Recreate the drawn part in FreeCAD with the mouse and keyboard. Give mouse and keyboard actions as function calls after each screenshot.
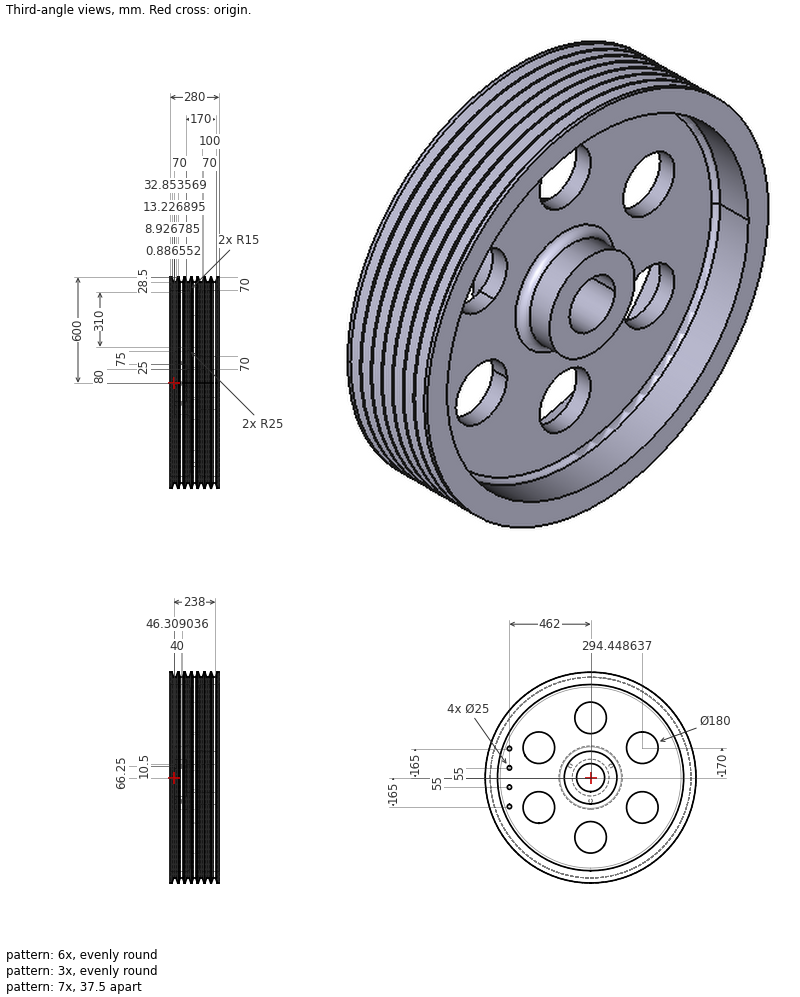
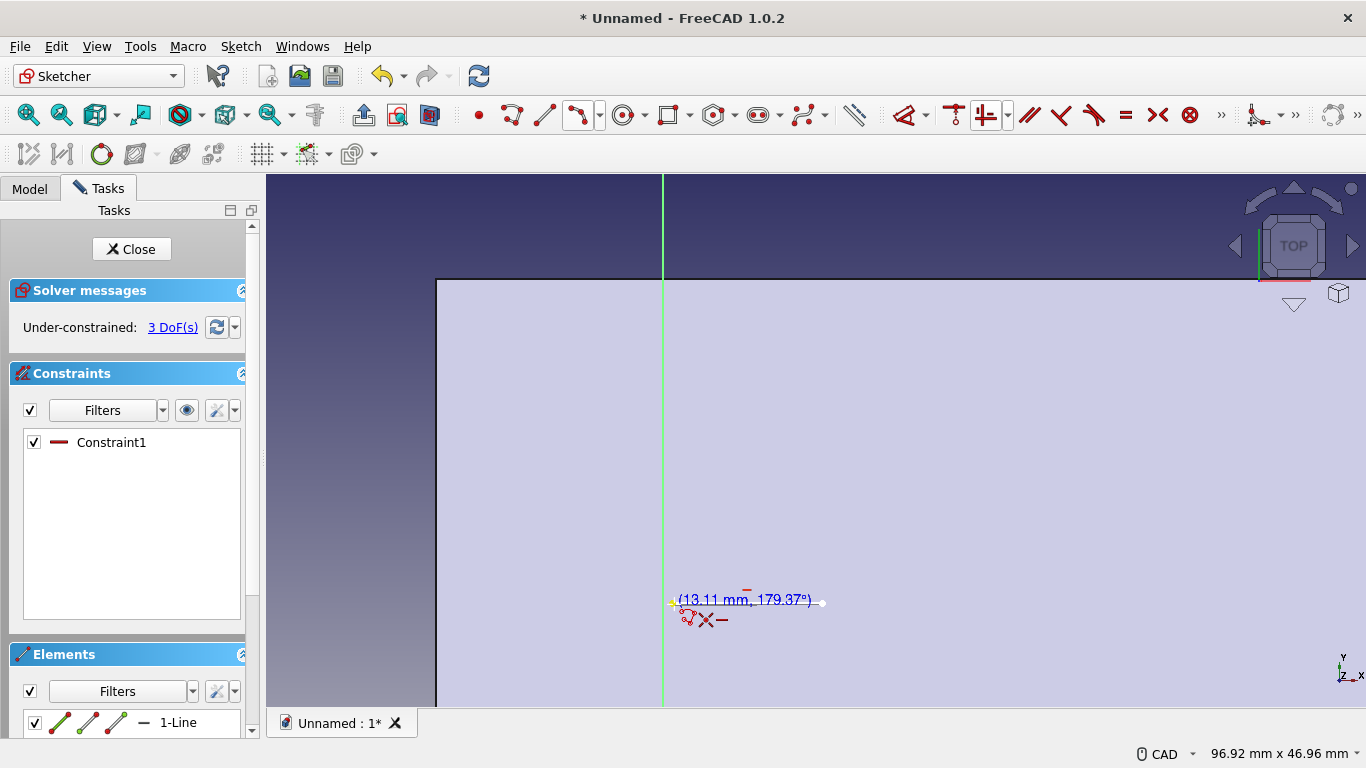
click(934, 279)
click(561, 279)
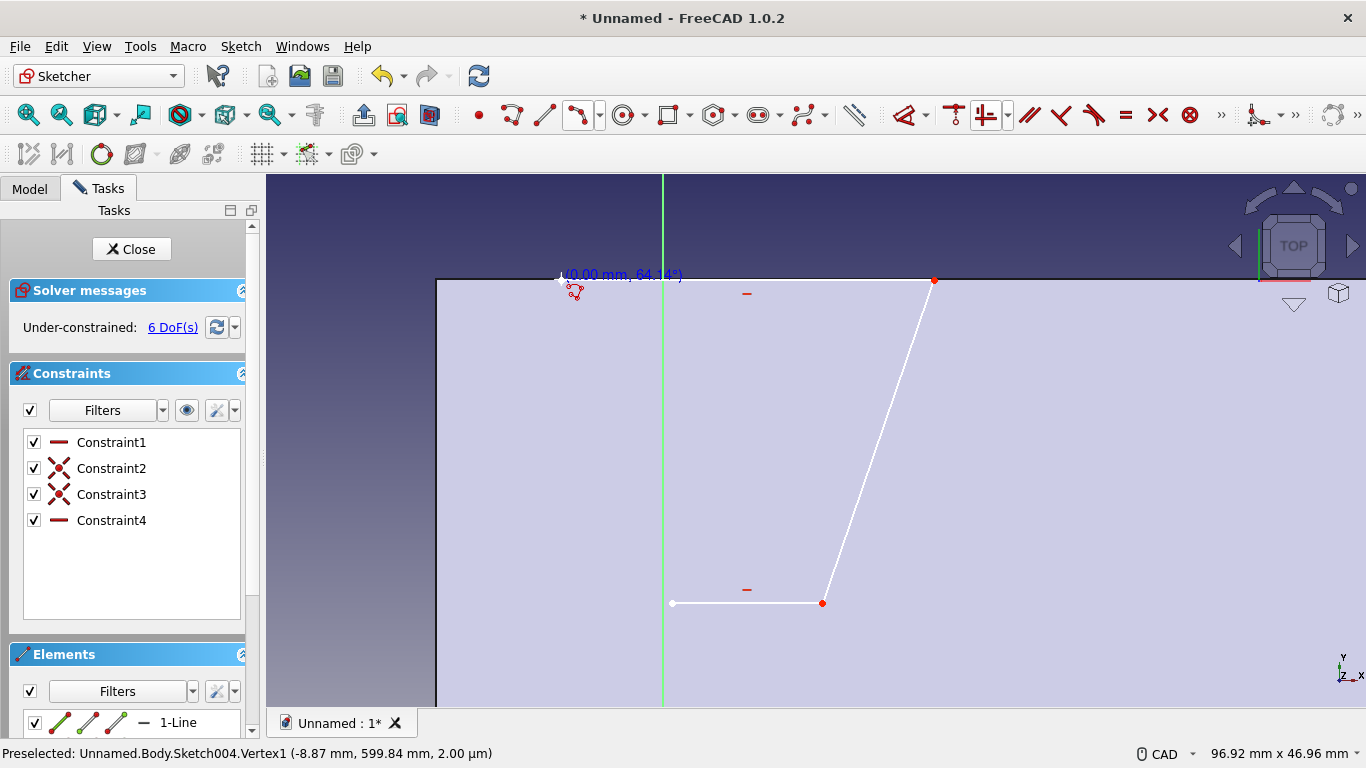
scroll(673, 603, up, 3)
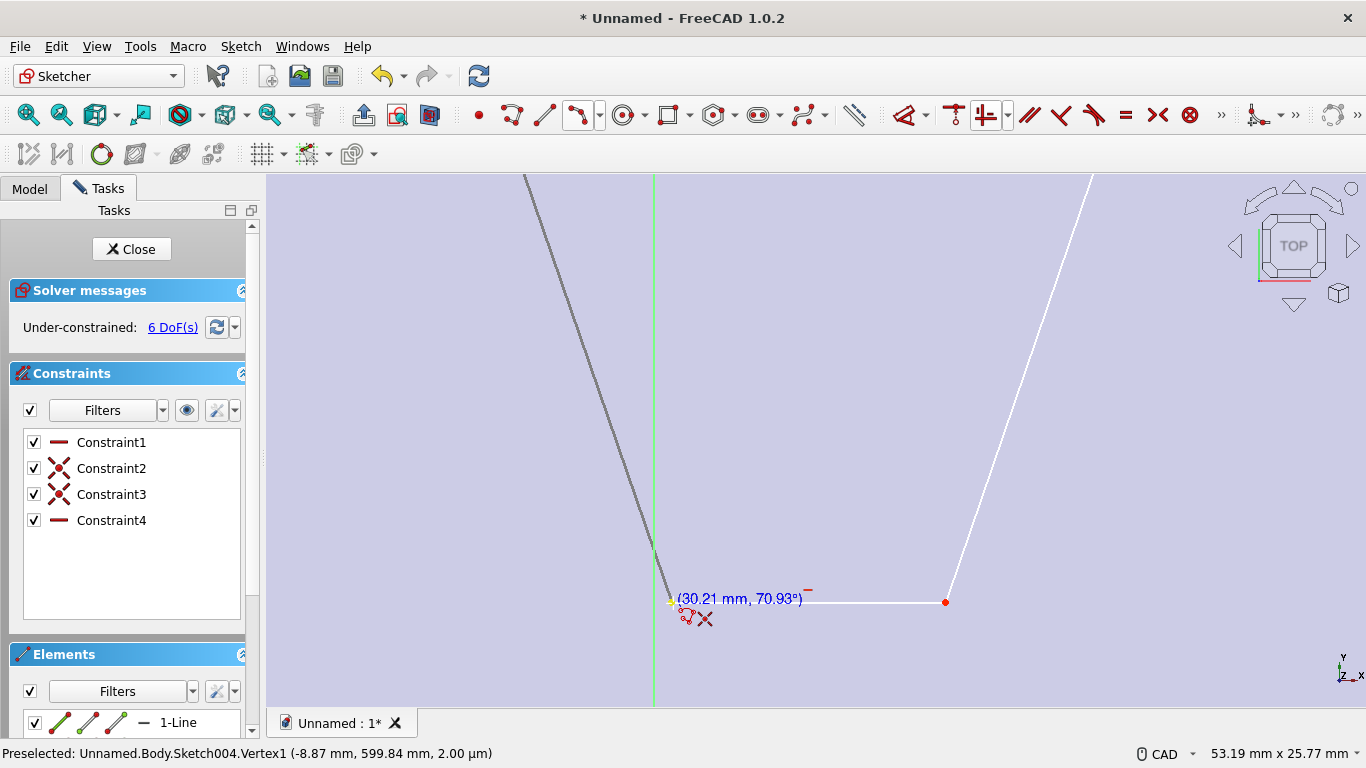
click(672, 603)
key(Escape)
key(Escape)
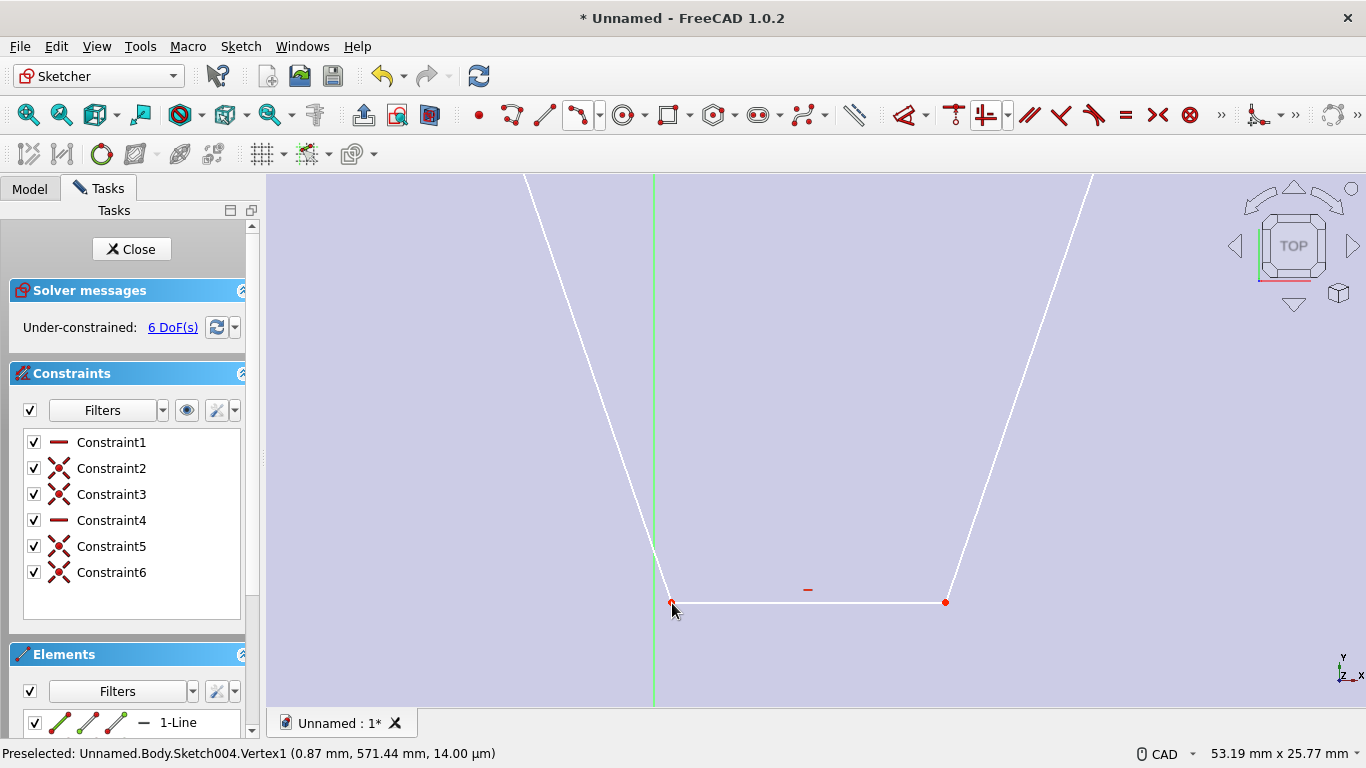
click(904, 116)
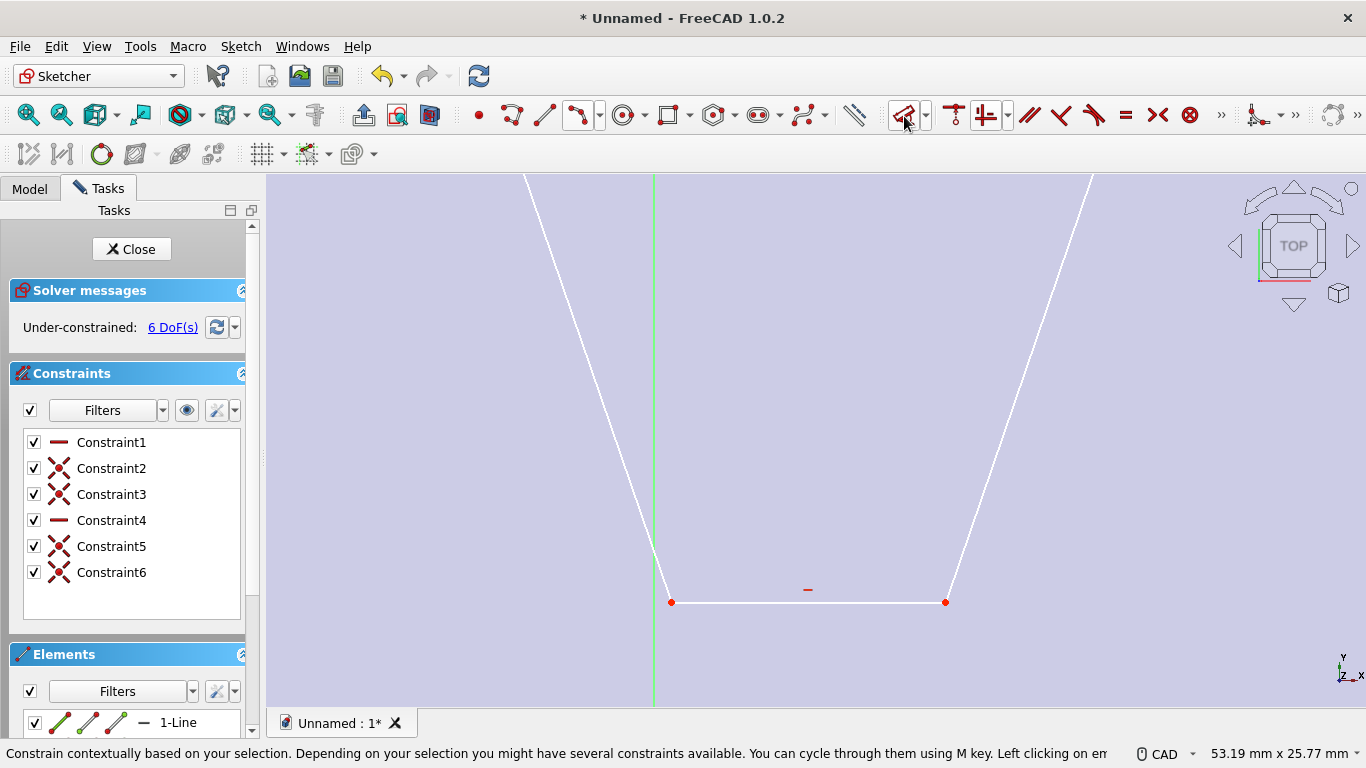
scroll(673, 603, down, 3)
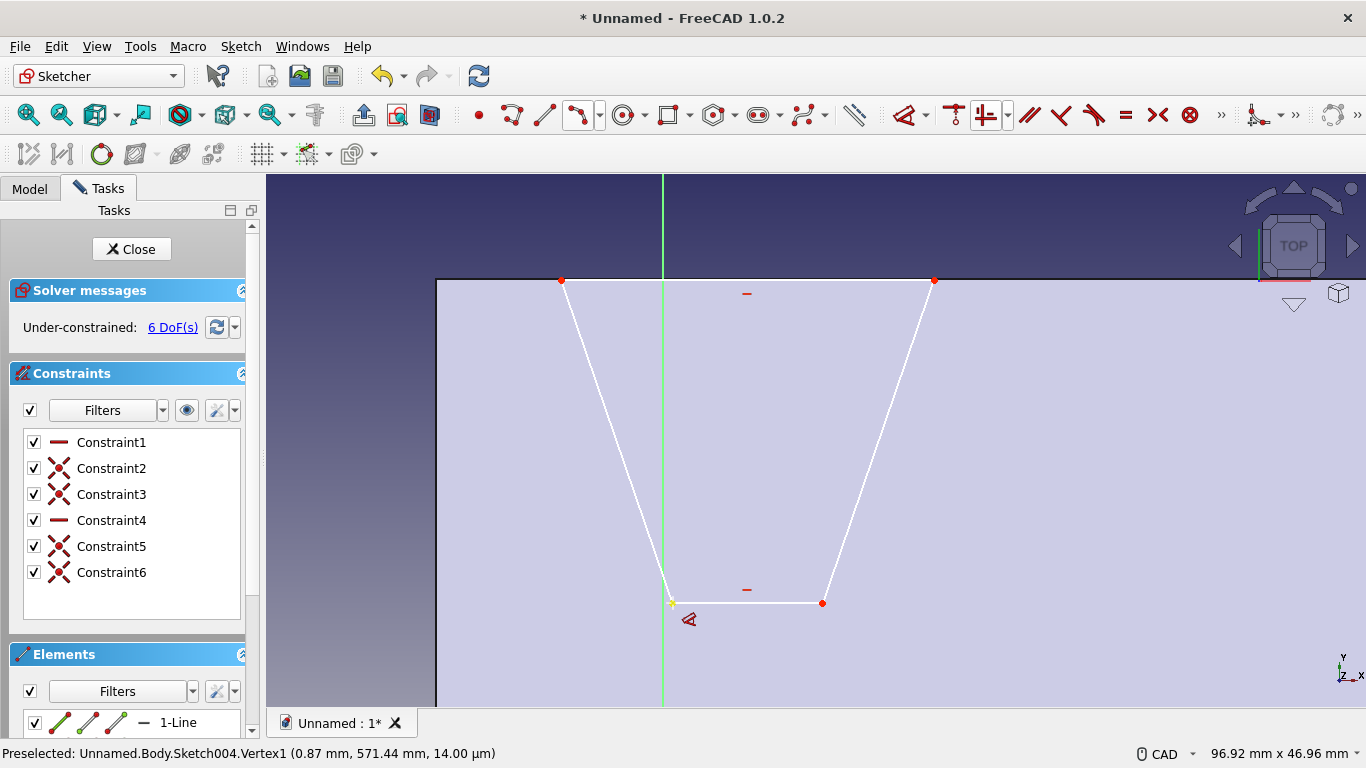
click(934, 280)
click(968, 480)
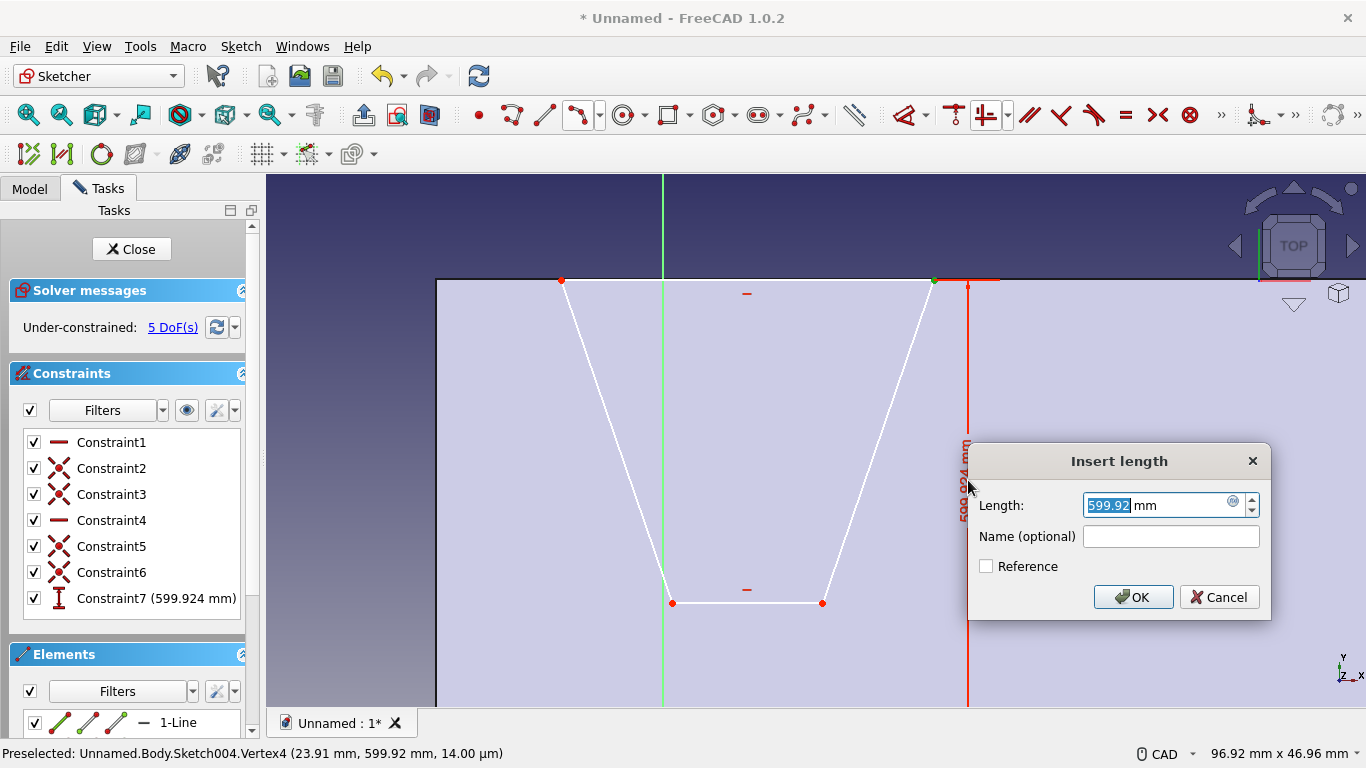
text(600)
key(Return)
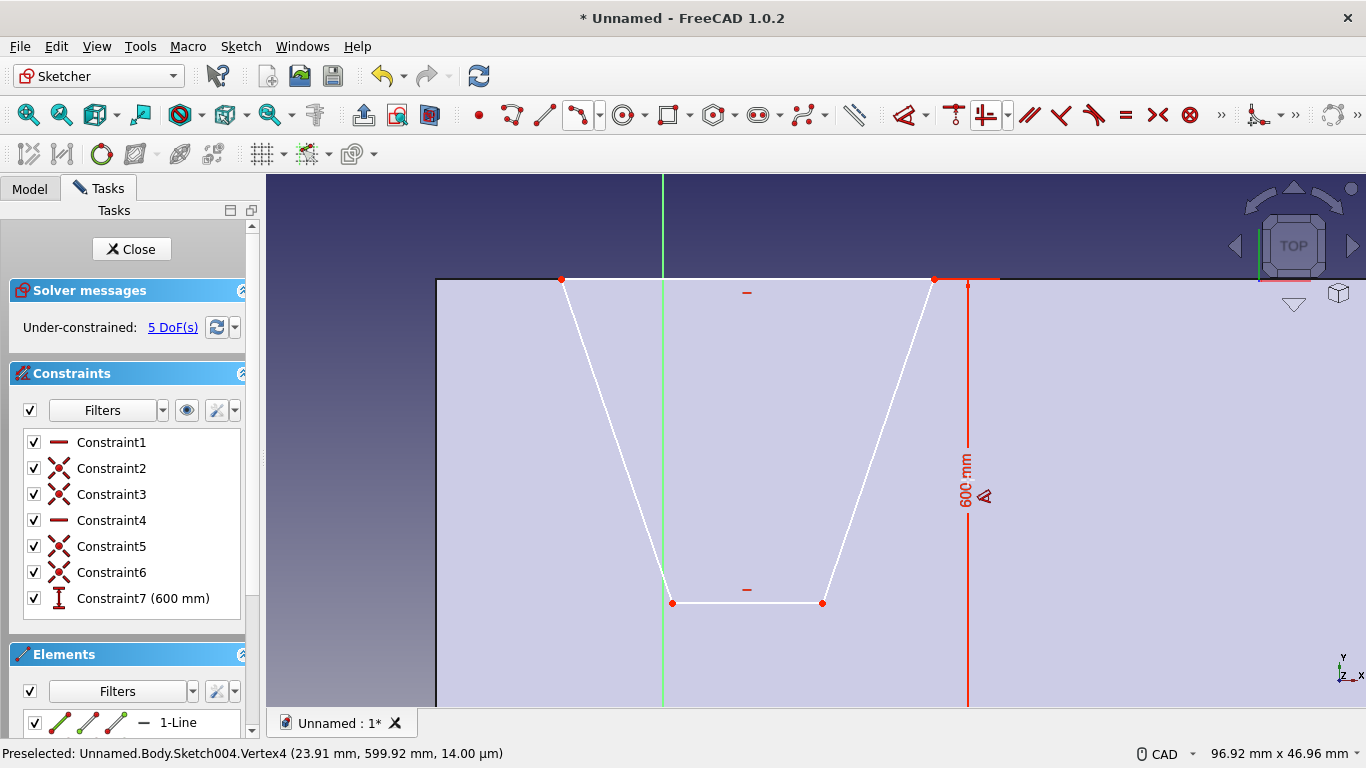
click(856, 506)
click(968, 441)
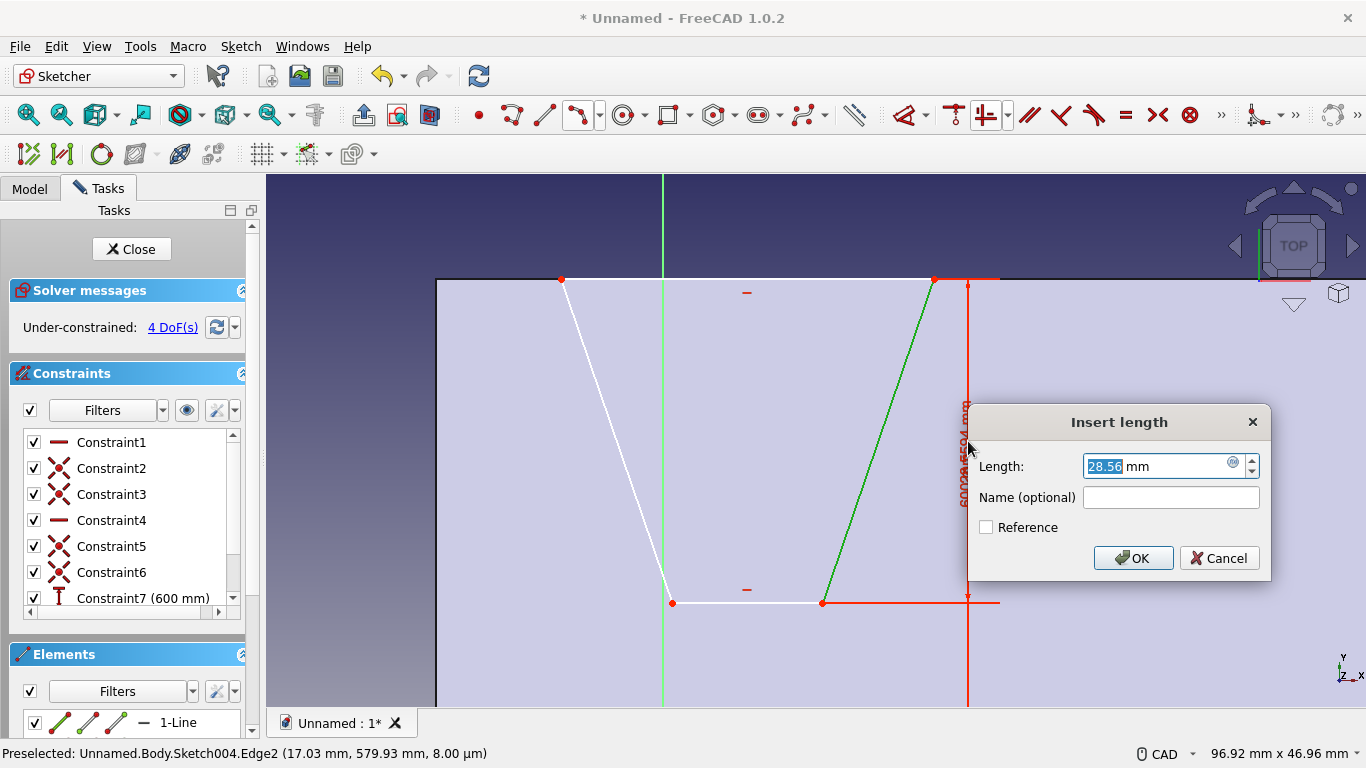
text(28.5)
key(Return)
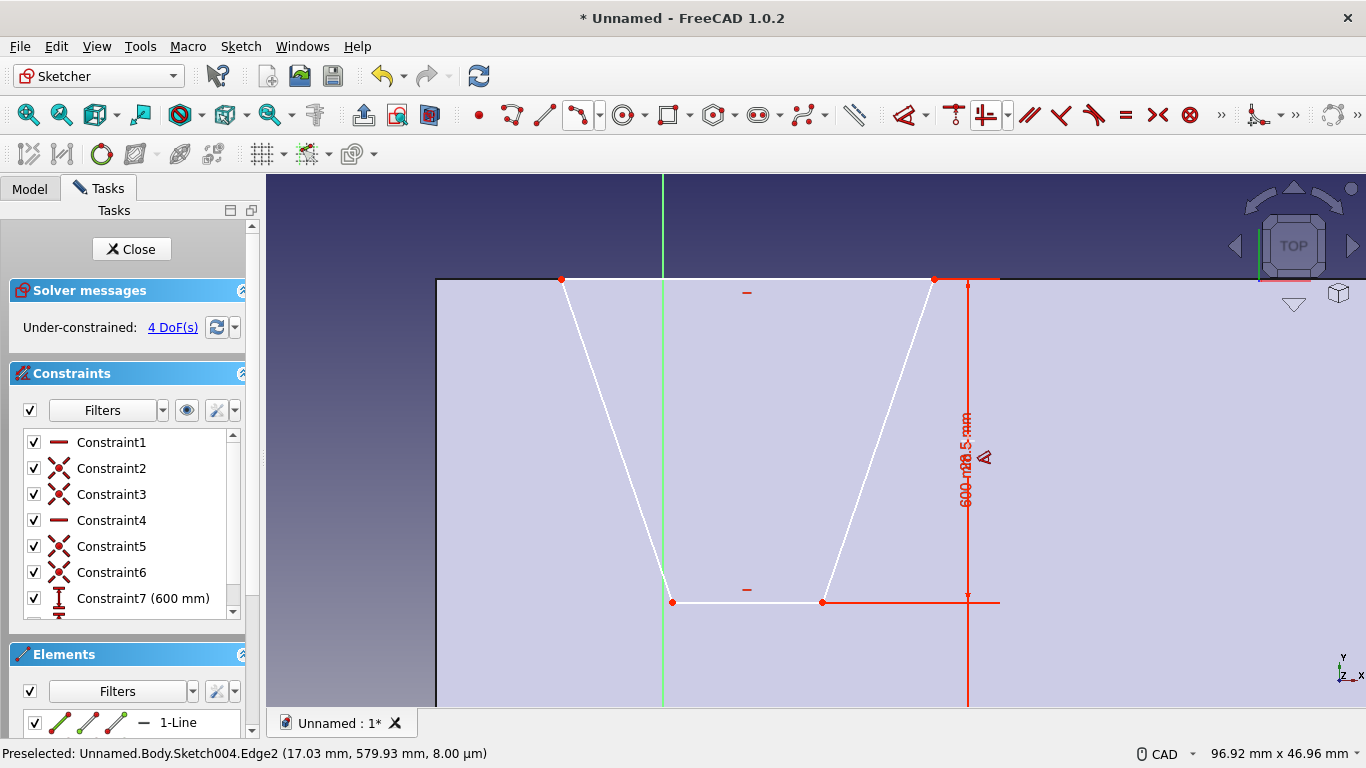
click(718, 603)
click(748, 637)